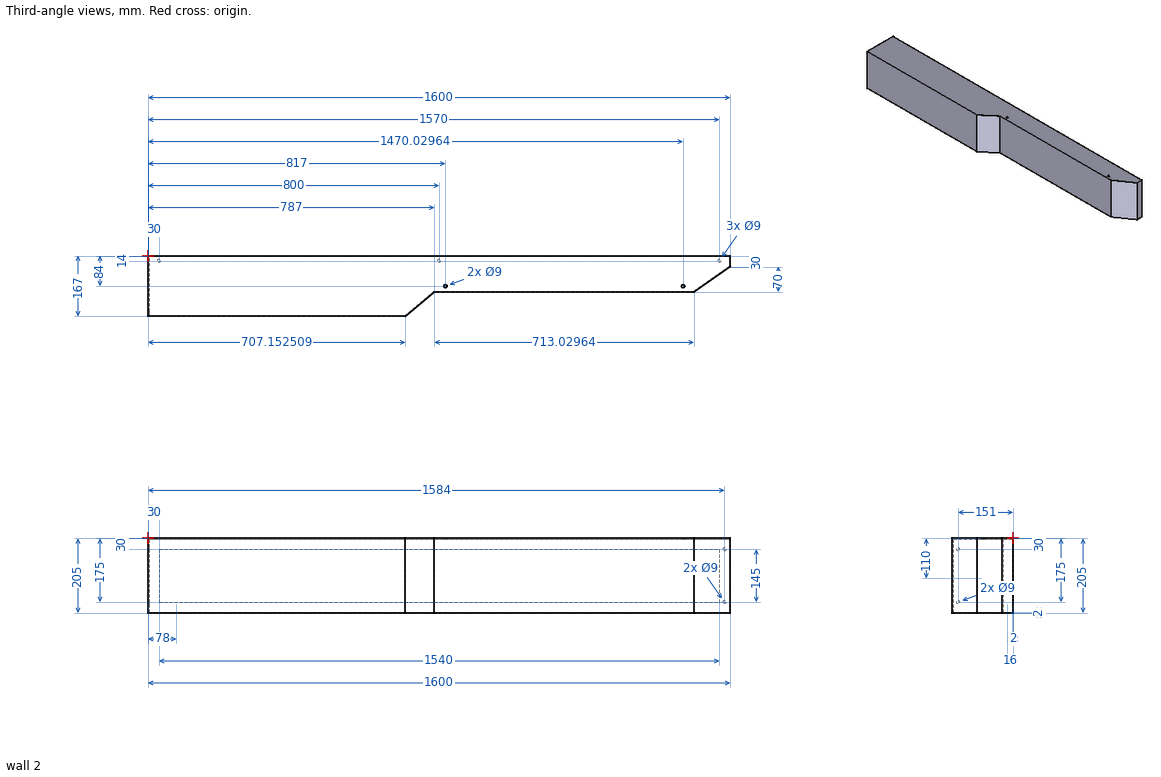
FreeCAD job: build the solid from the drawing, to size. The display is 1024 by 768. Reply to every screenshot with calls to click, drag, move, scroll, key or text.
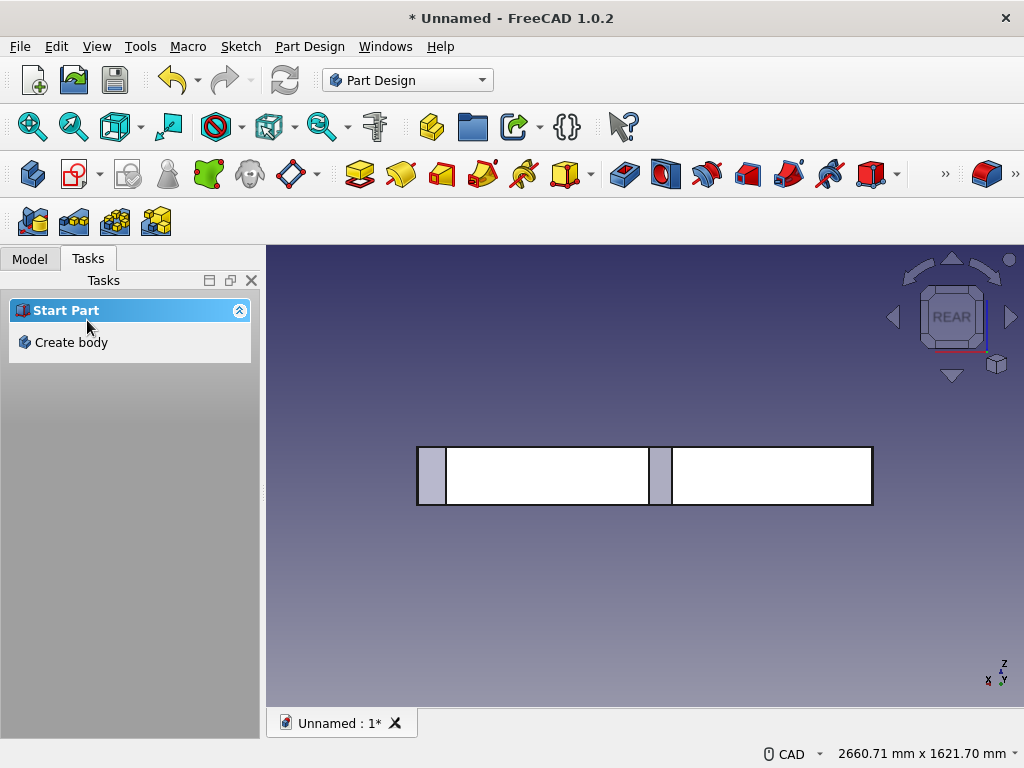
scroll(417, 465, up, 15)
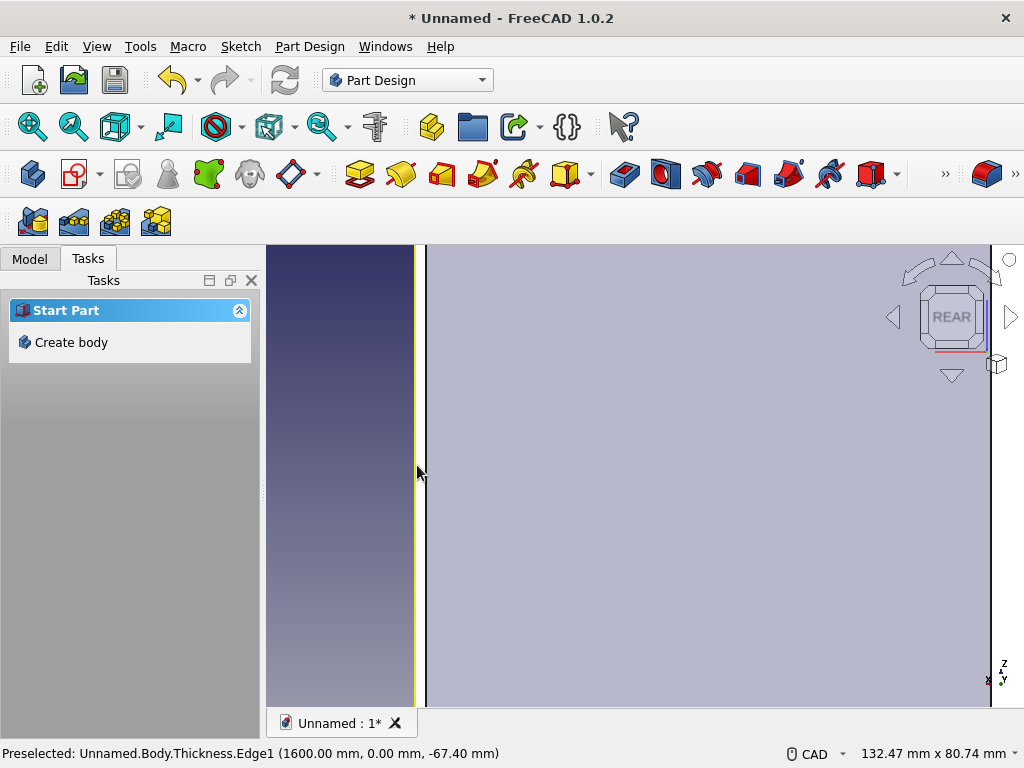
scroll(419, 484, up, 6)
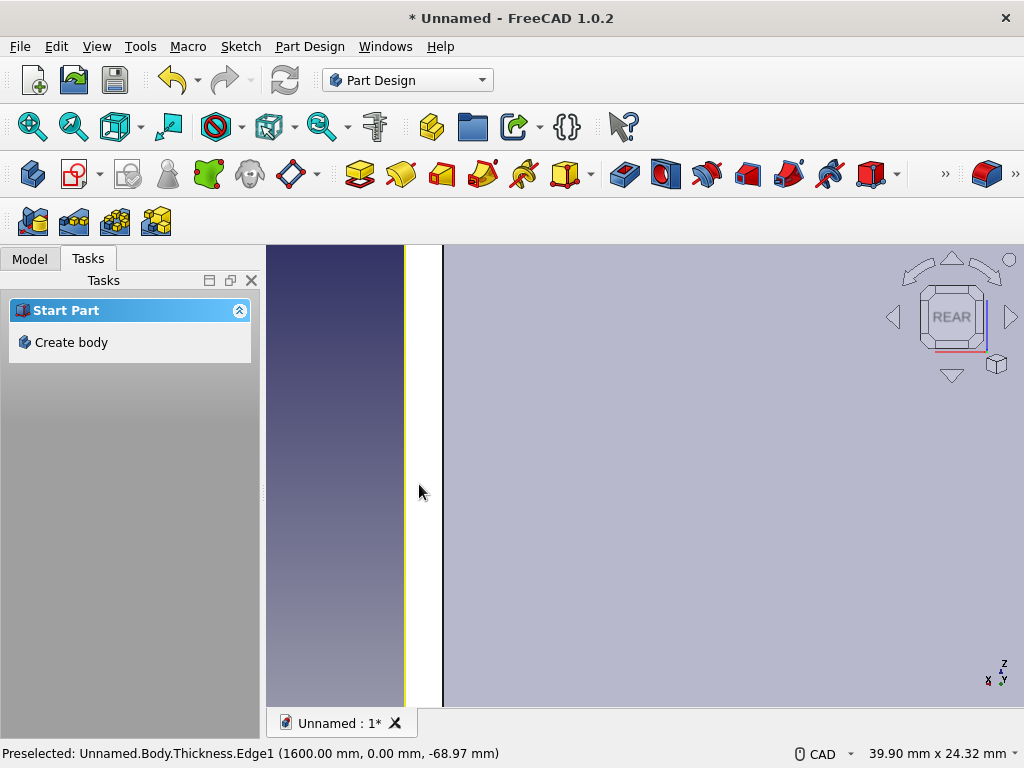
click(418, 486)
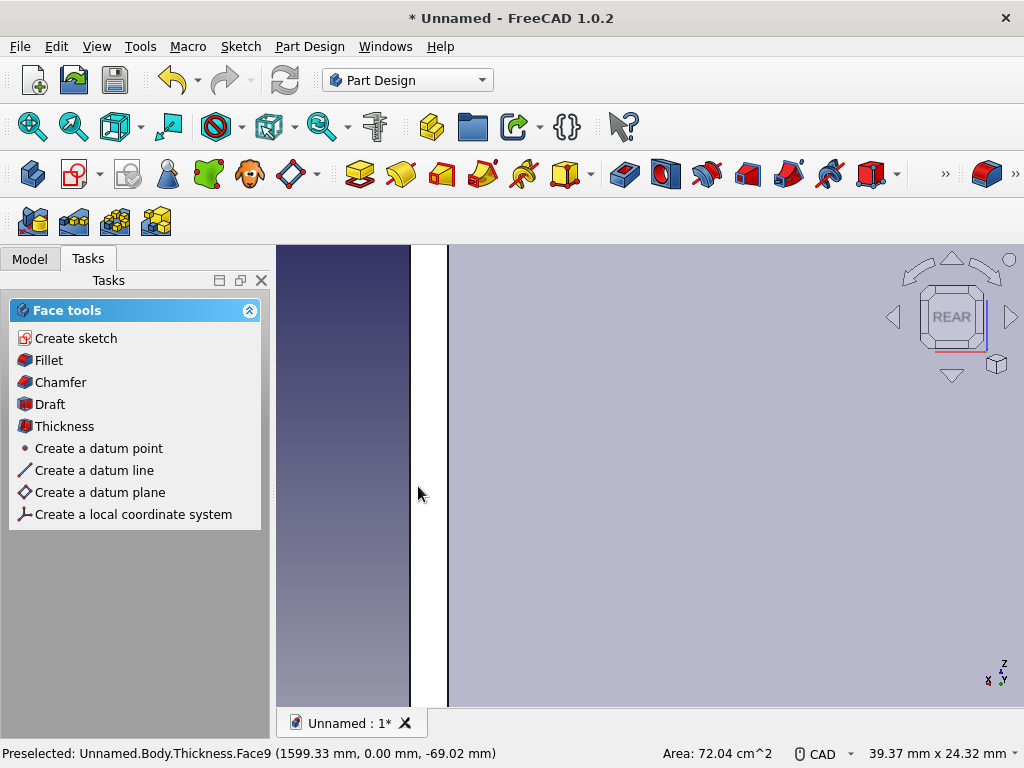
click(74, 174)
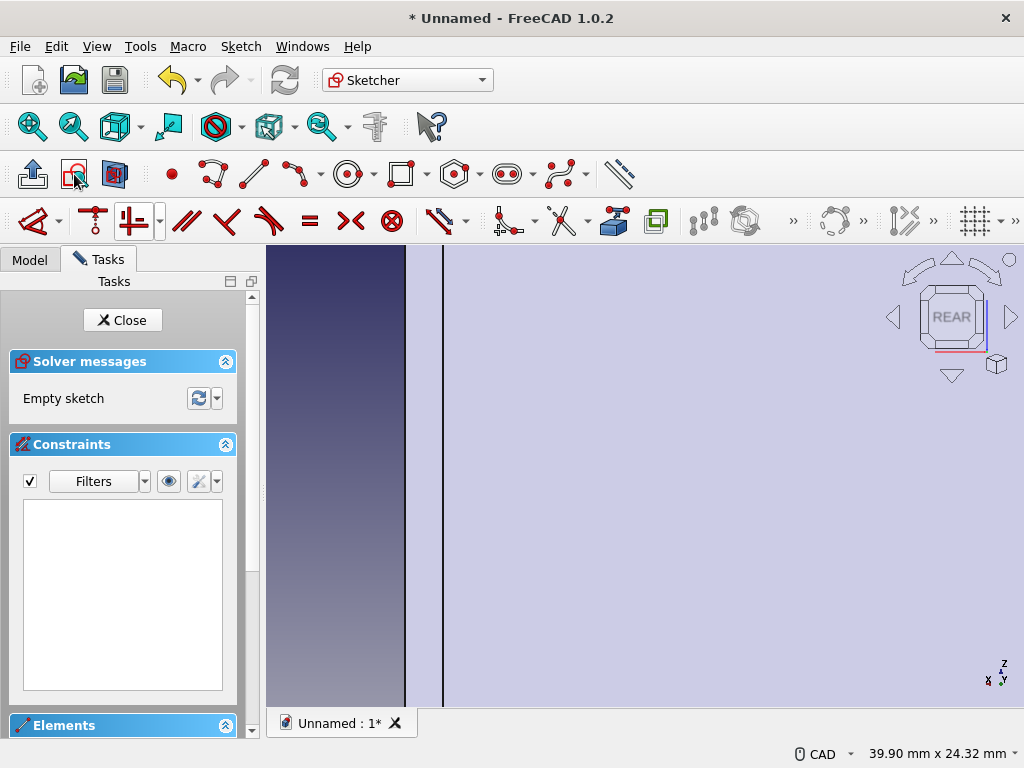
scroll(576, 476, down, 15)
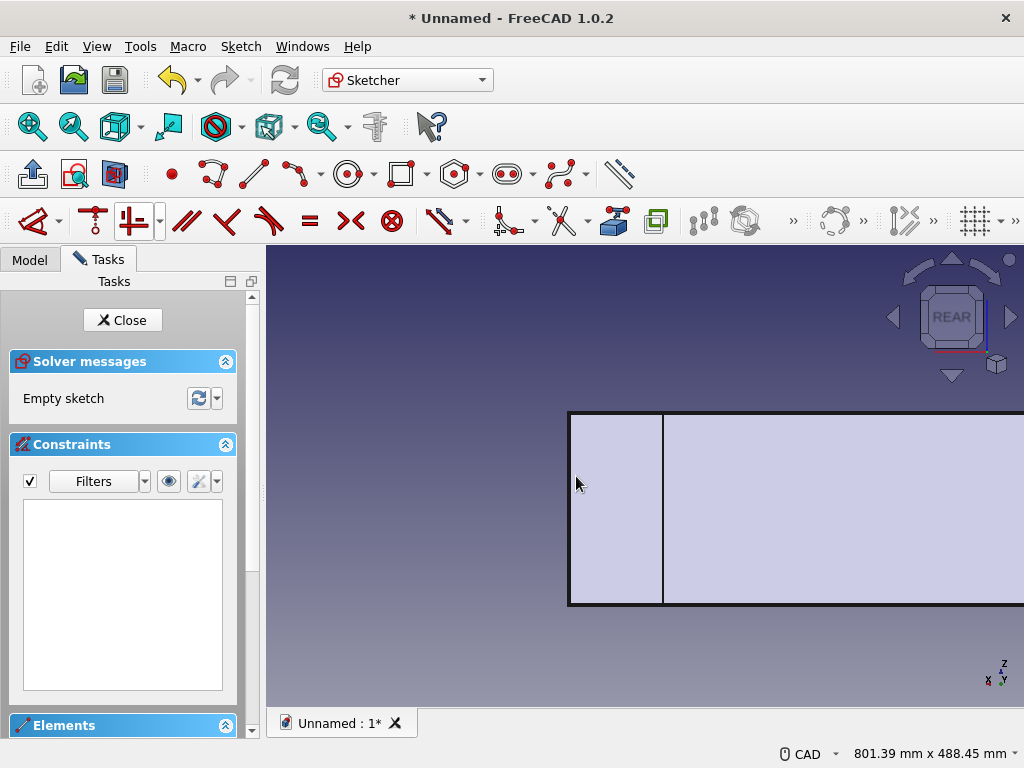
scroll(332, 465, down, 7)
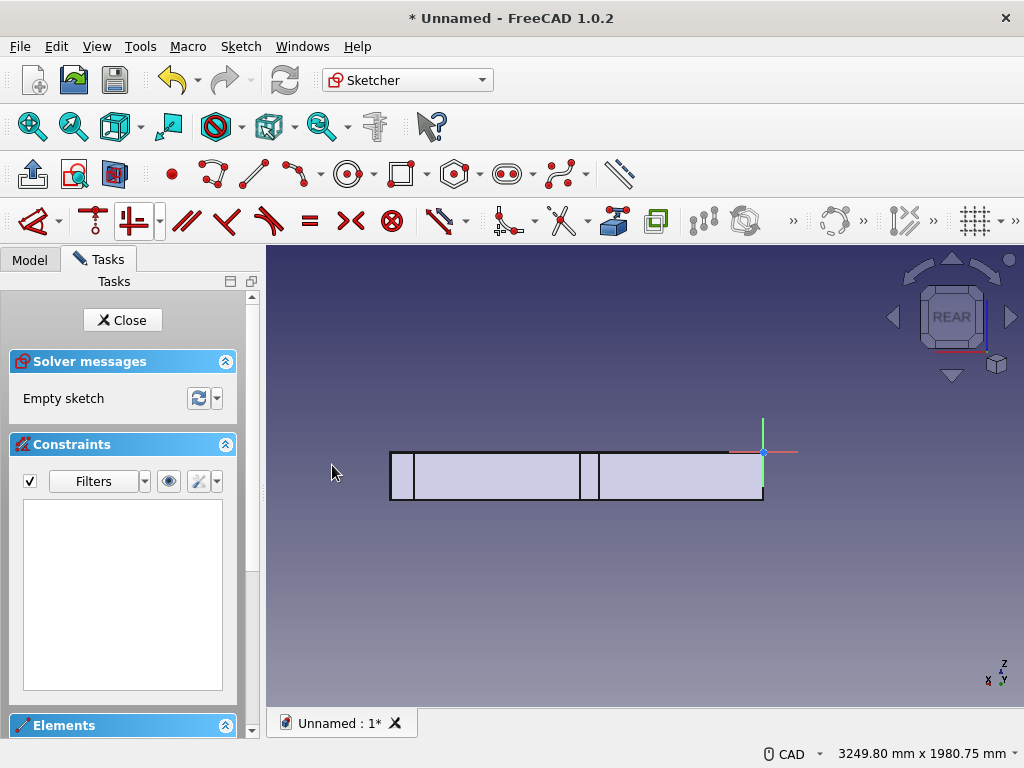
key(g)
key(r)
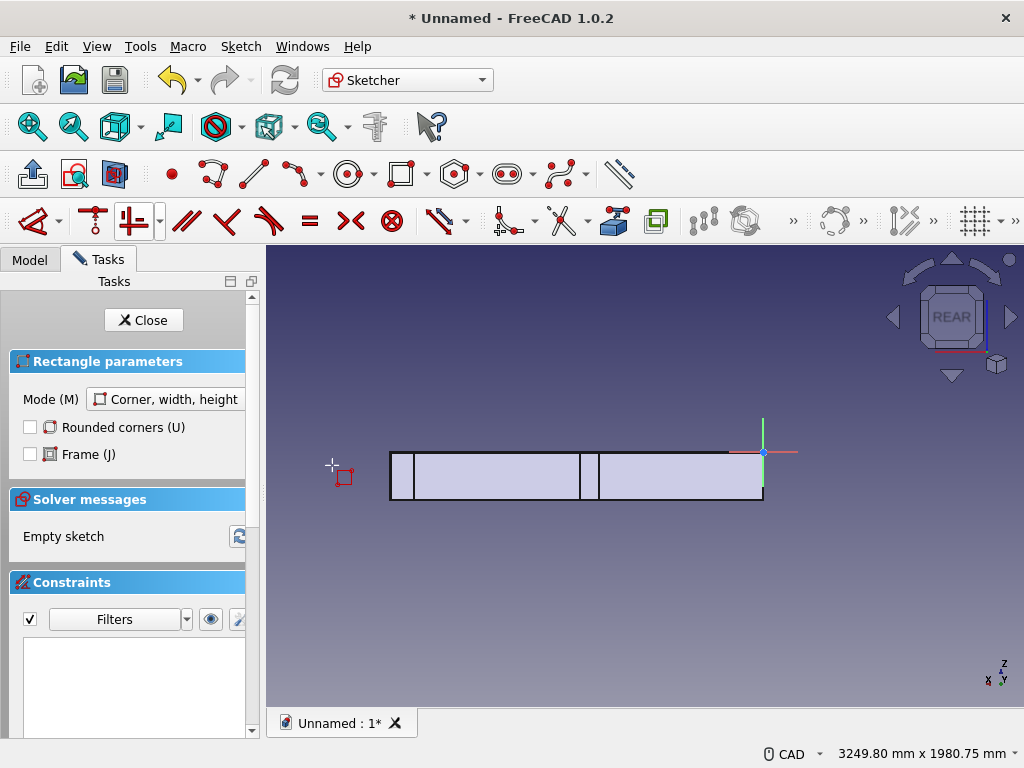
click(763, 452)
move(390, 500)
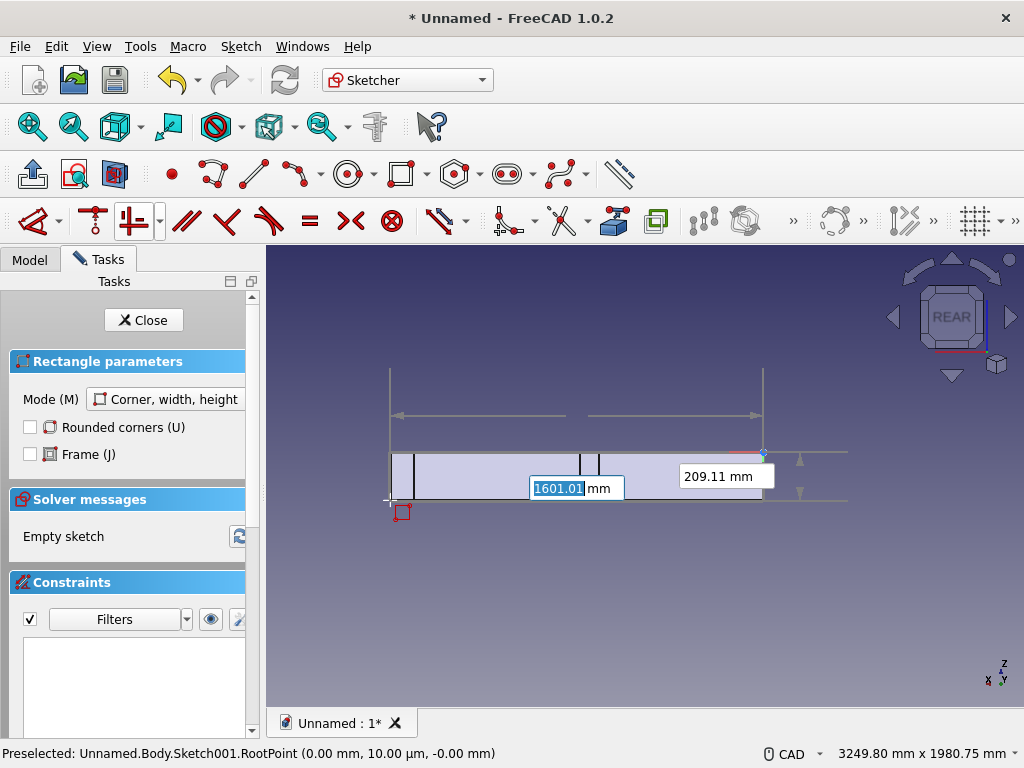
text(1600)
key(Tab)
text(205)
key(Return)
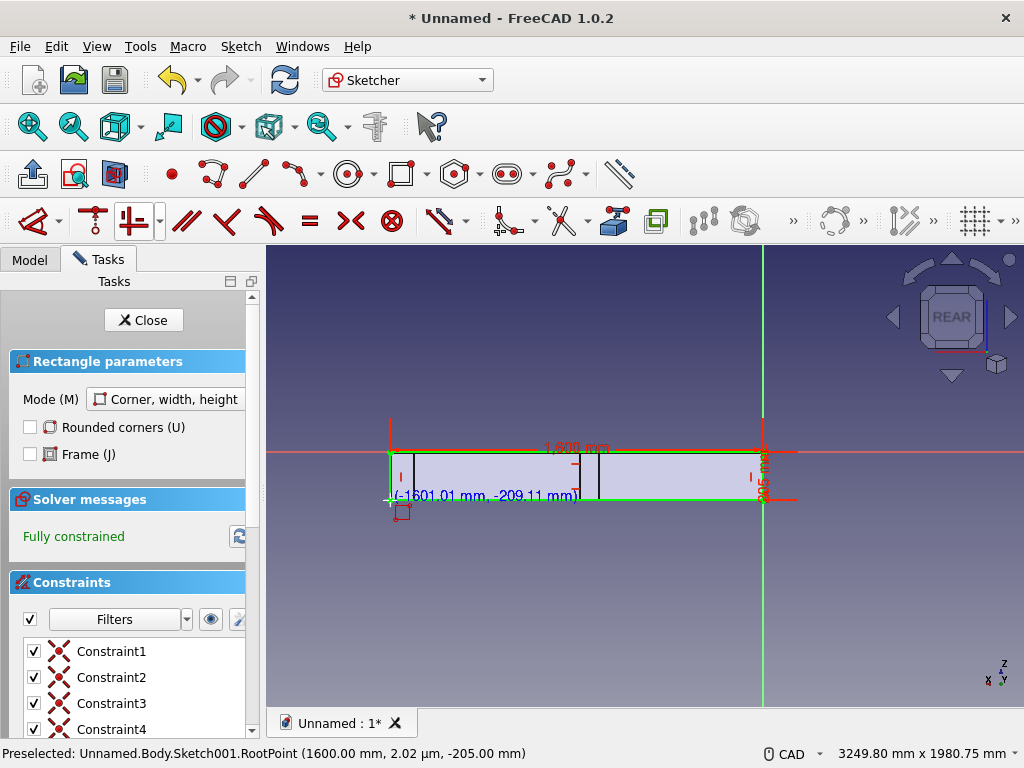
scroll(397, 459, up, 5)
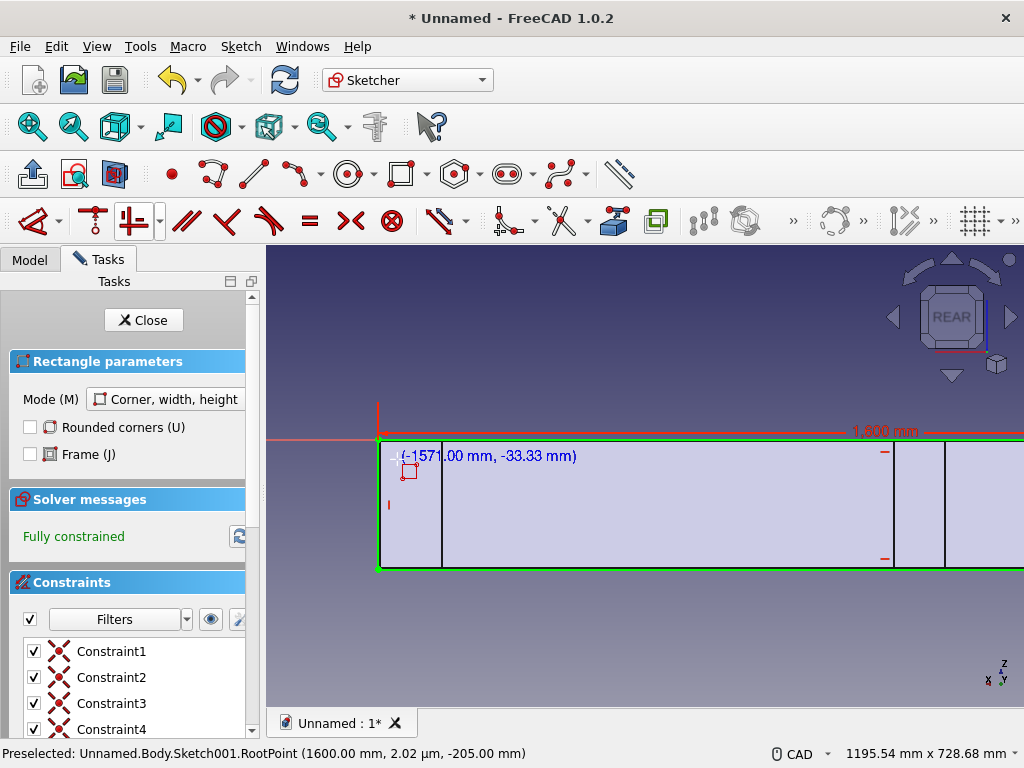
click(397, 459)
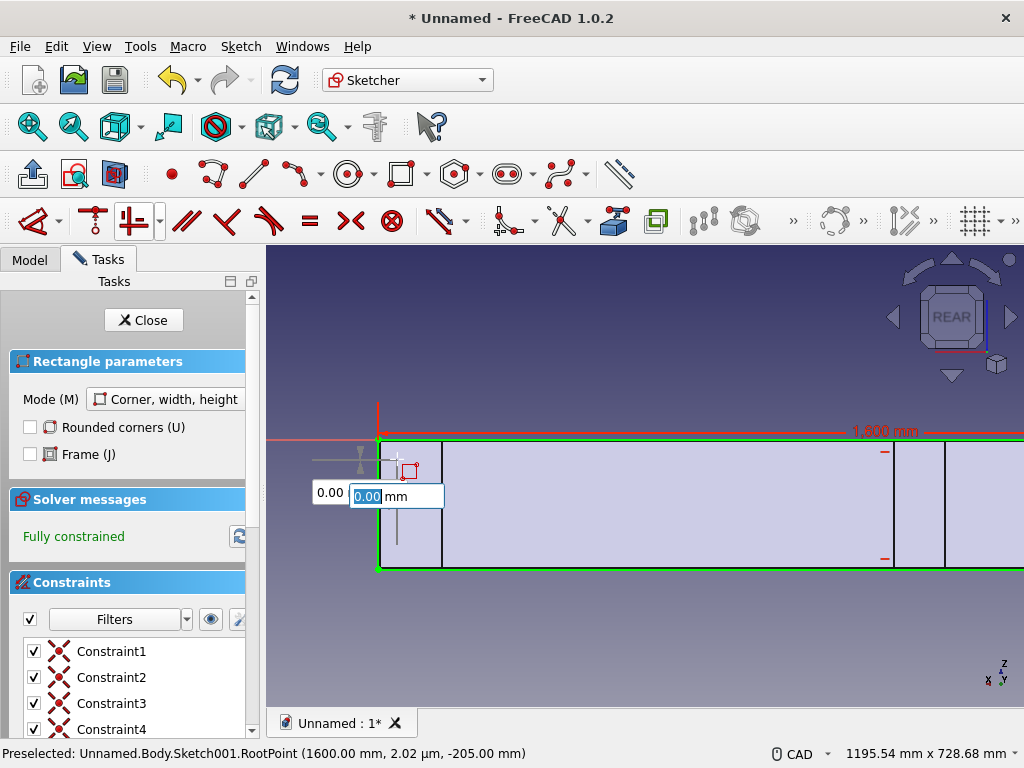
scroll(397, 459, down, 5)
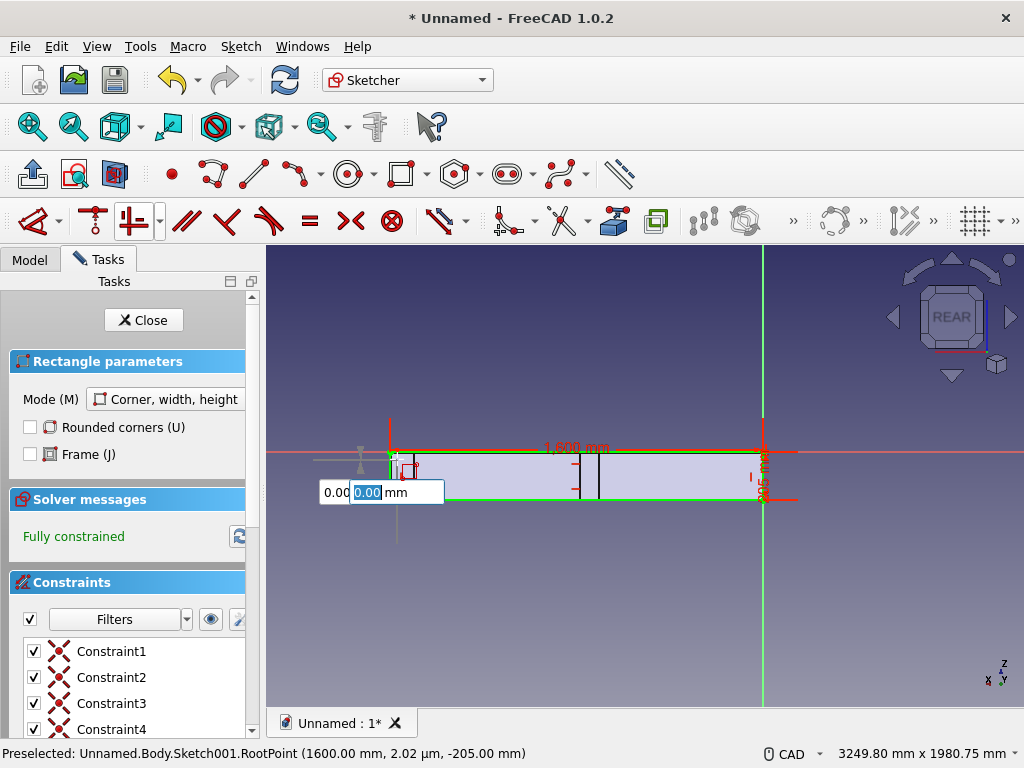
scroll(756, 493, up, 5)